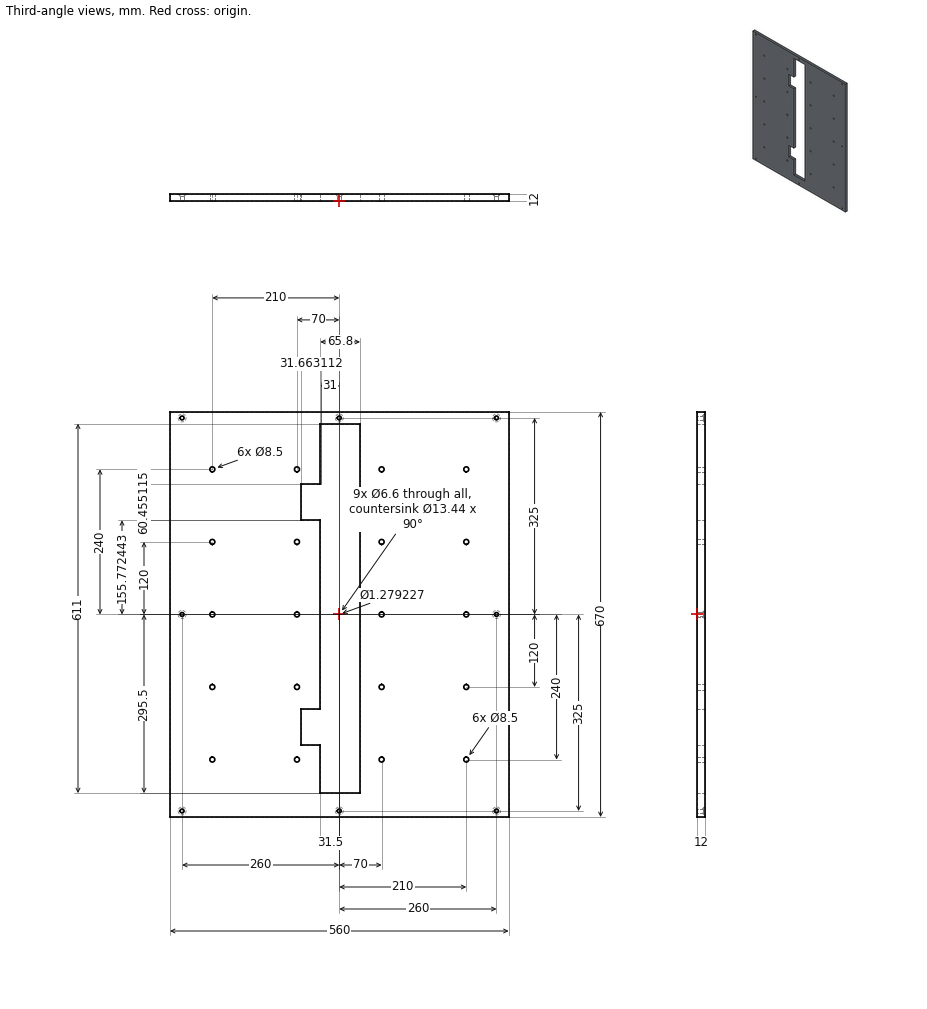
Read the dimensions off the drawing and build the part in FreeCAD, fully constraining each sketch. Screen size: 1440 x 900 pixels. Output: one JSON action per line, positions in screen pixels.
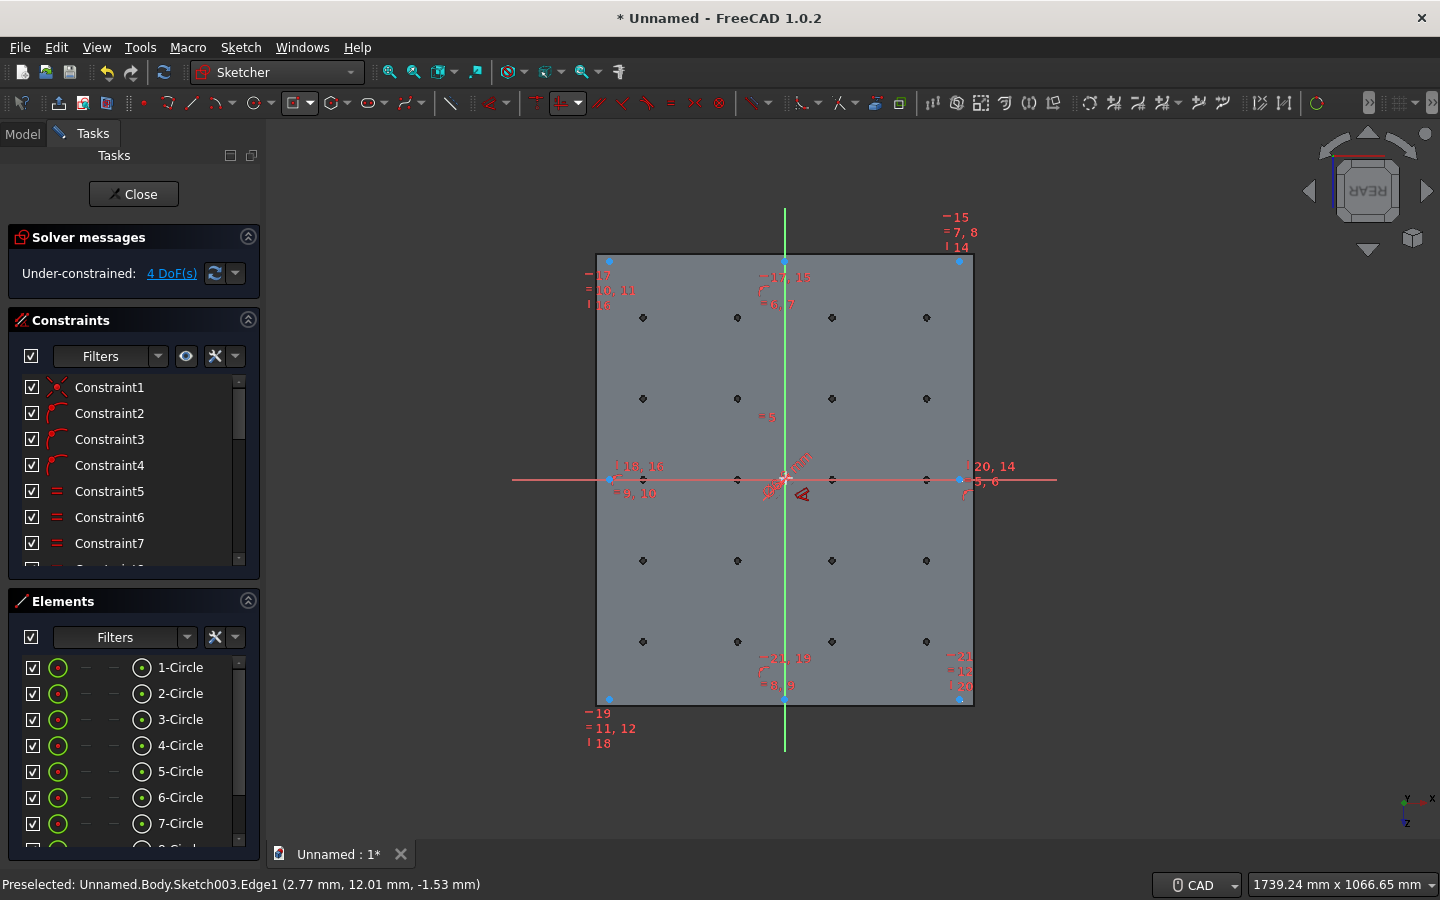
{"action": "left_click", "coordinate": [960, 480]}
{"action": "left_click", "coordinate": [872, 514]}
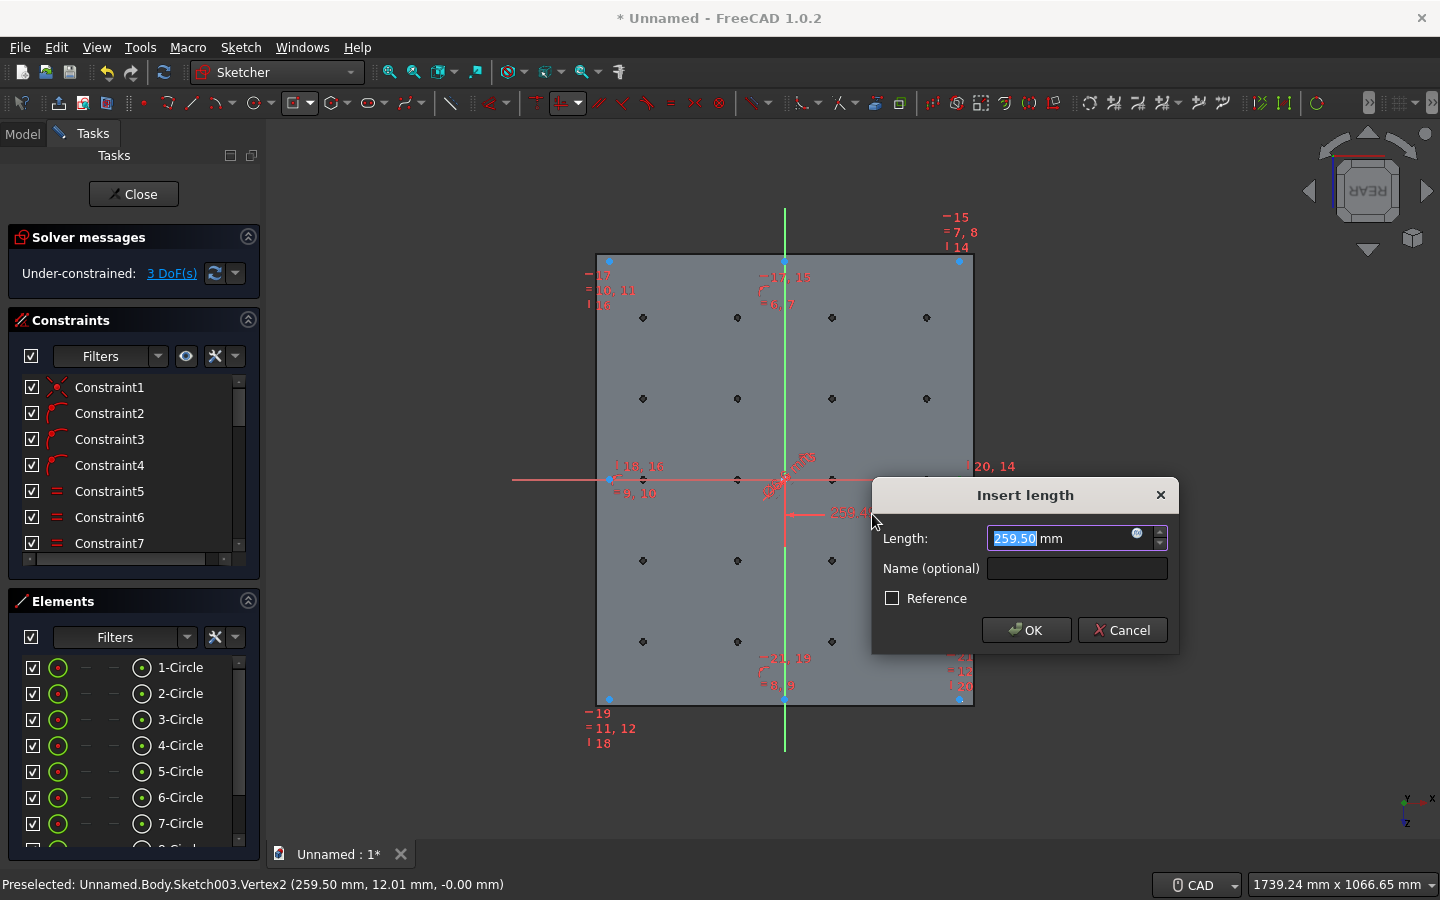
{"action": "type", "text": "260"}
{"action": "key", "text": "Return"}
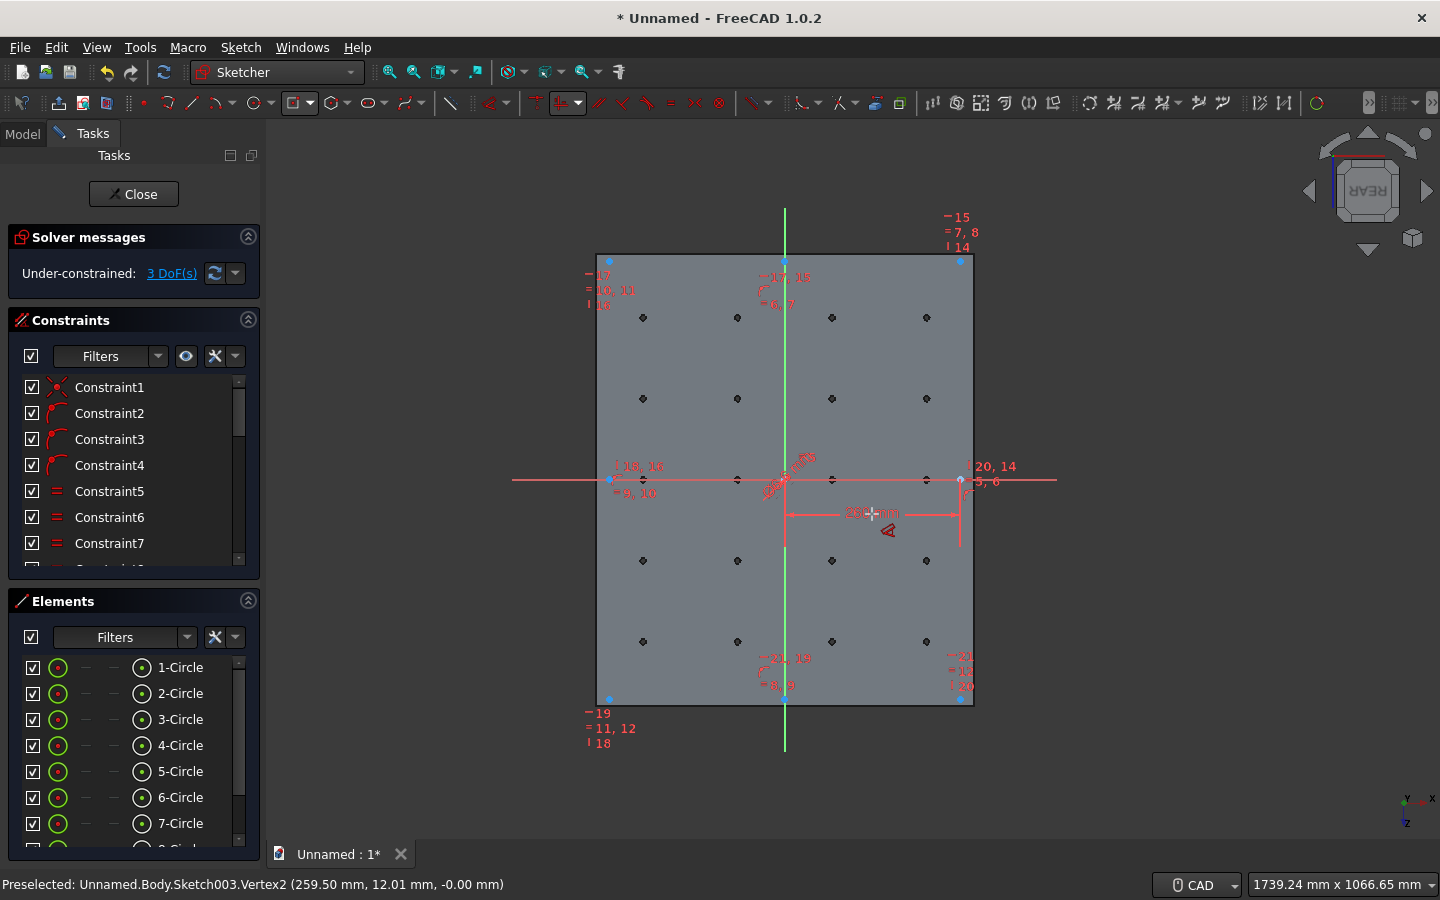
{"action": "left_click", "coordinate": [785, 262]}
{"action": "left_click", "coordinate": [819, 371]}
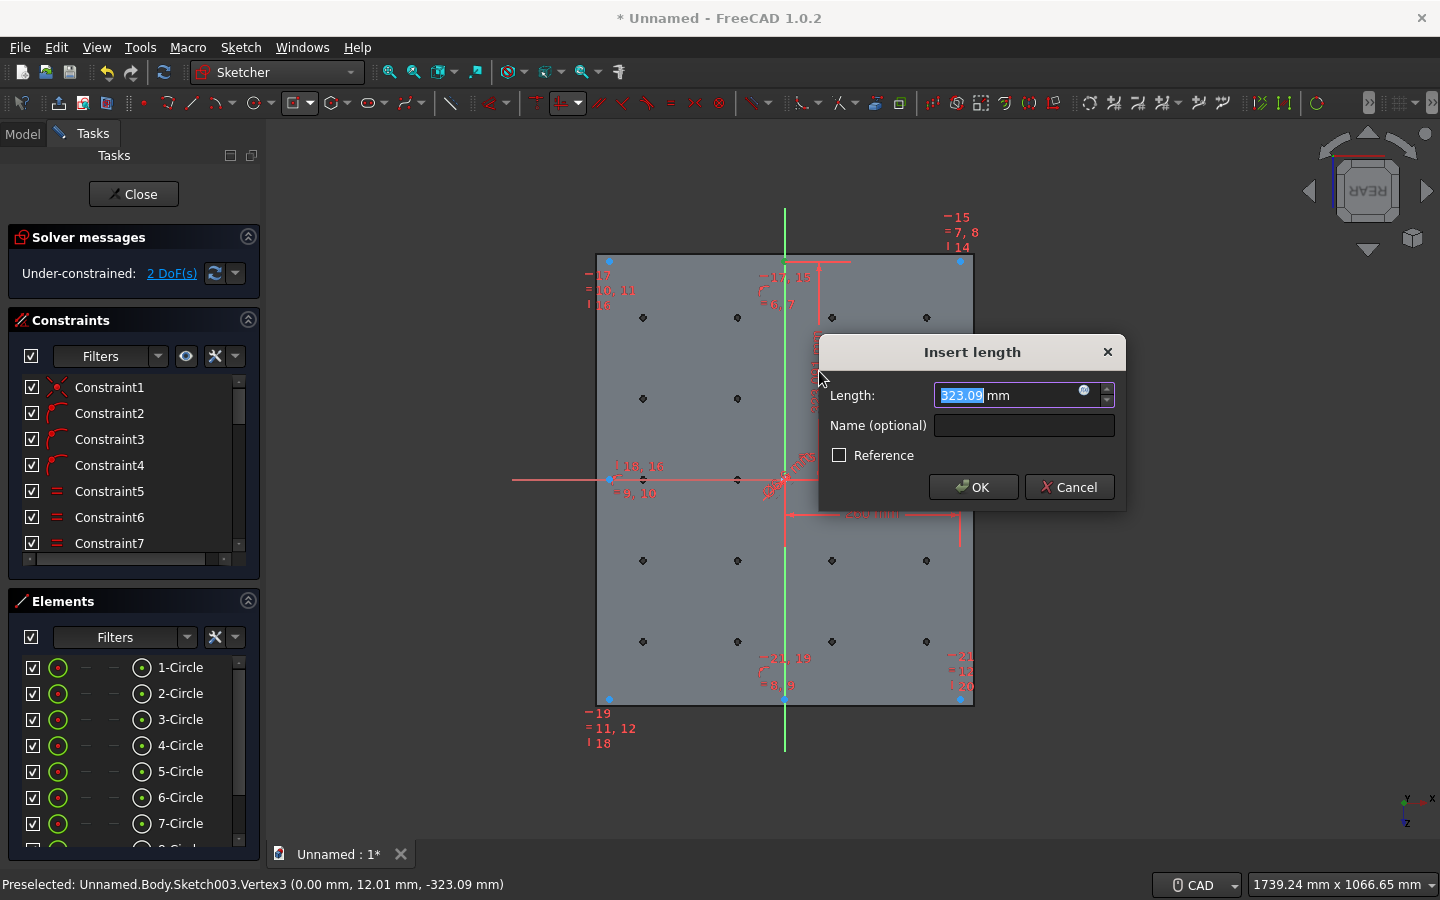
{"action": "type", "text": "325"}
{"action": "key", "text": "Return"}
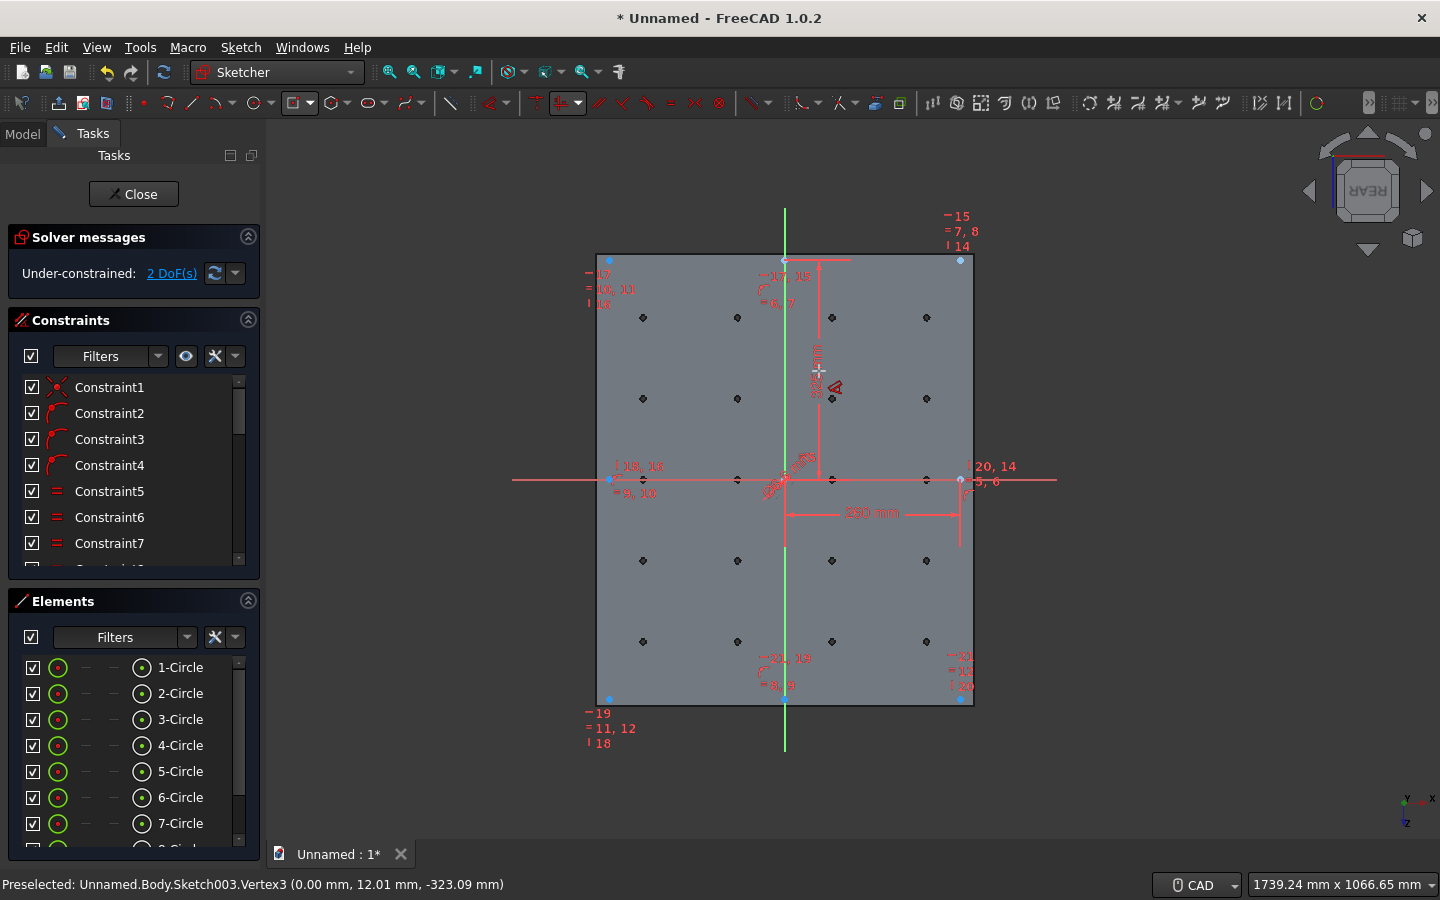
{"action": "left_click", "coordinate": [785, 700]}
{"action": "left_click", "coordinate": [819, 590]}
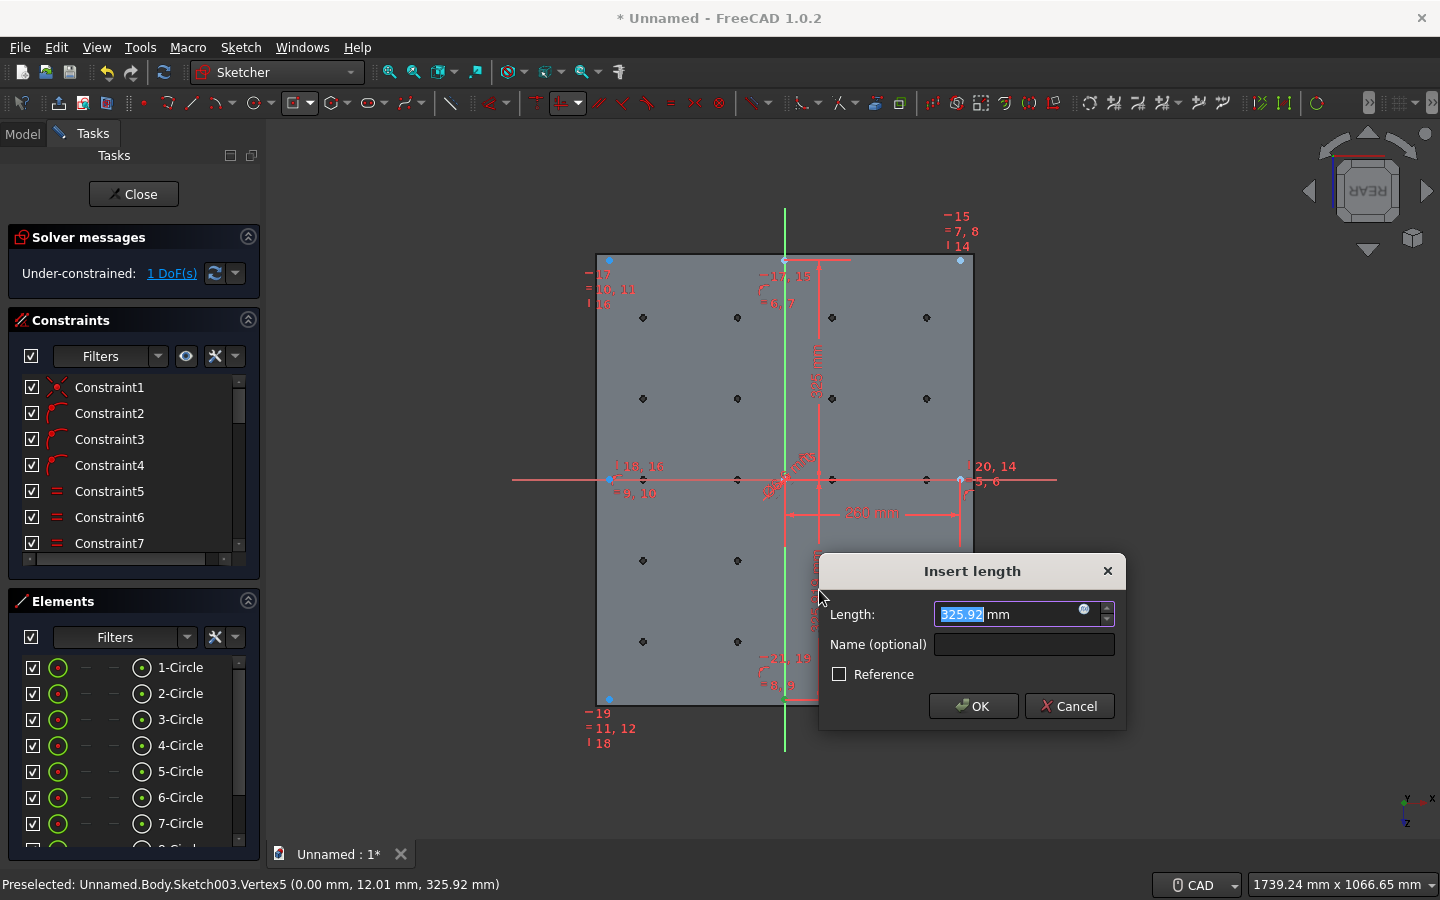
{"action": "type", "text": "325"}
{"action": "key", "text": "Return"}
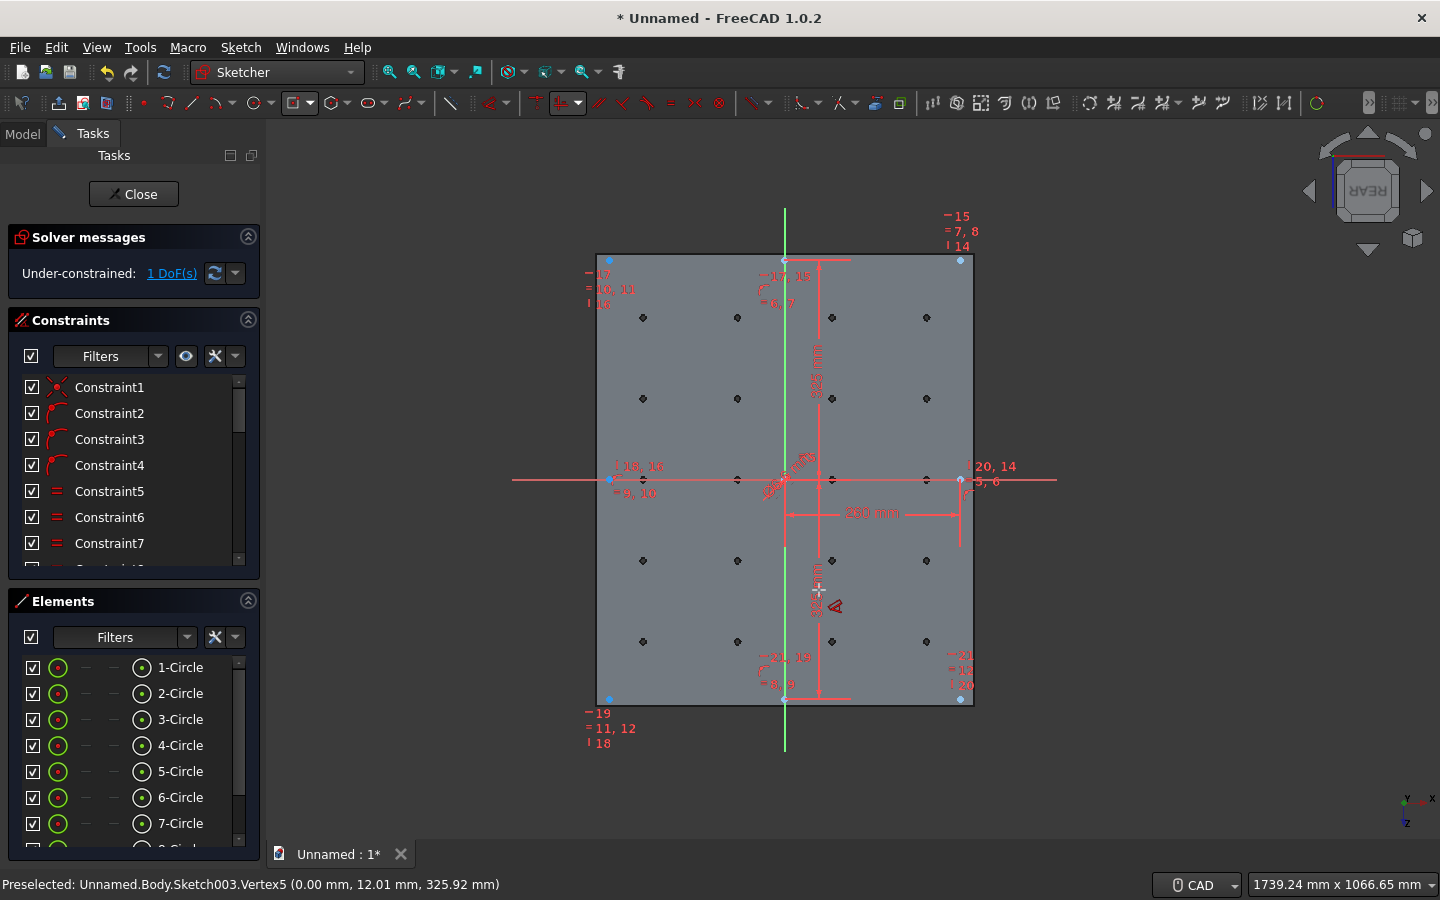
{"action": "left_click", "coordinate": [609, 480]}
{"action": "left_click", "coordinate": [697, 514]}